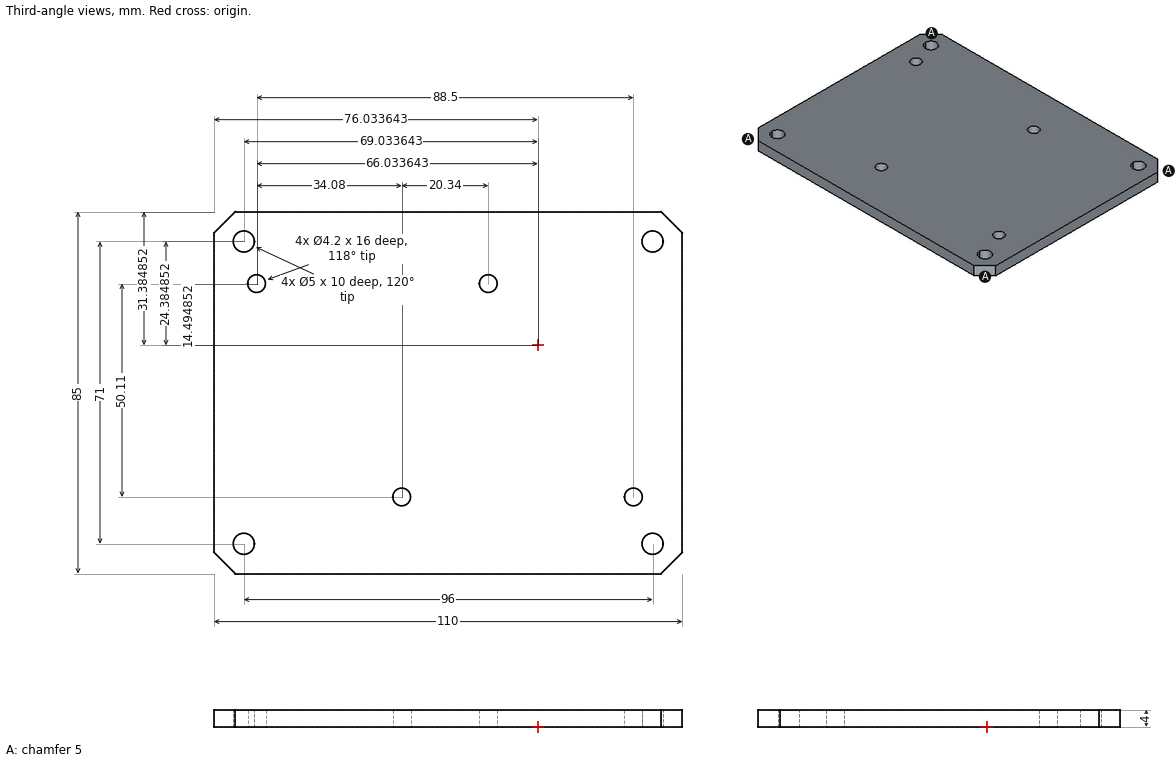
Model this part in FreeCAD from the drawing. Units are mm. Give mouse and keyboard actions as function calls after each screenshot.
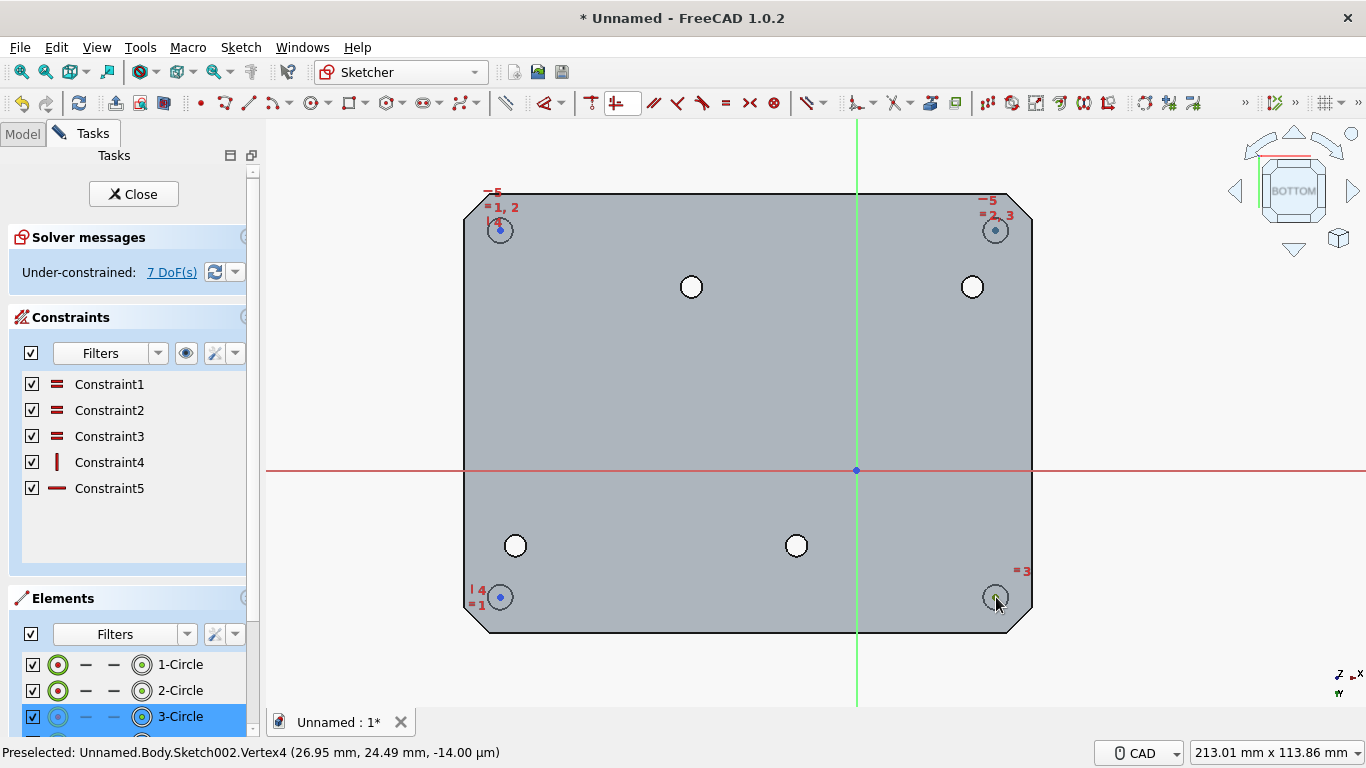
key(v)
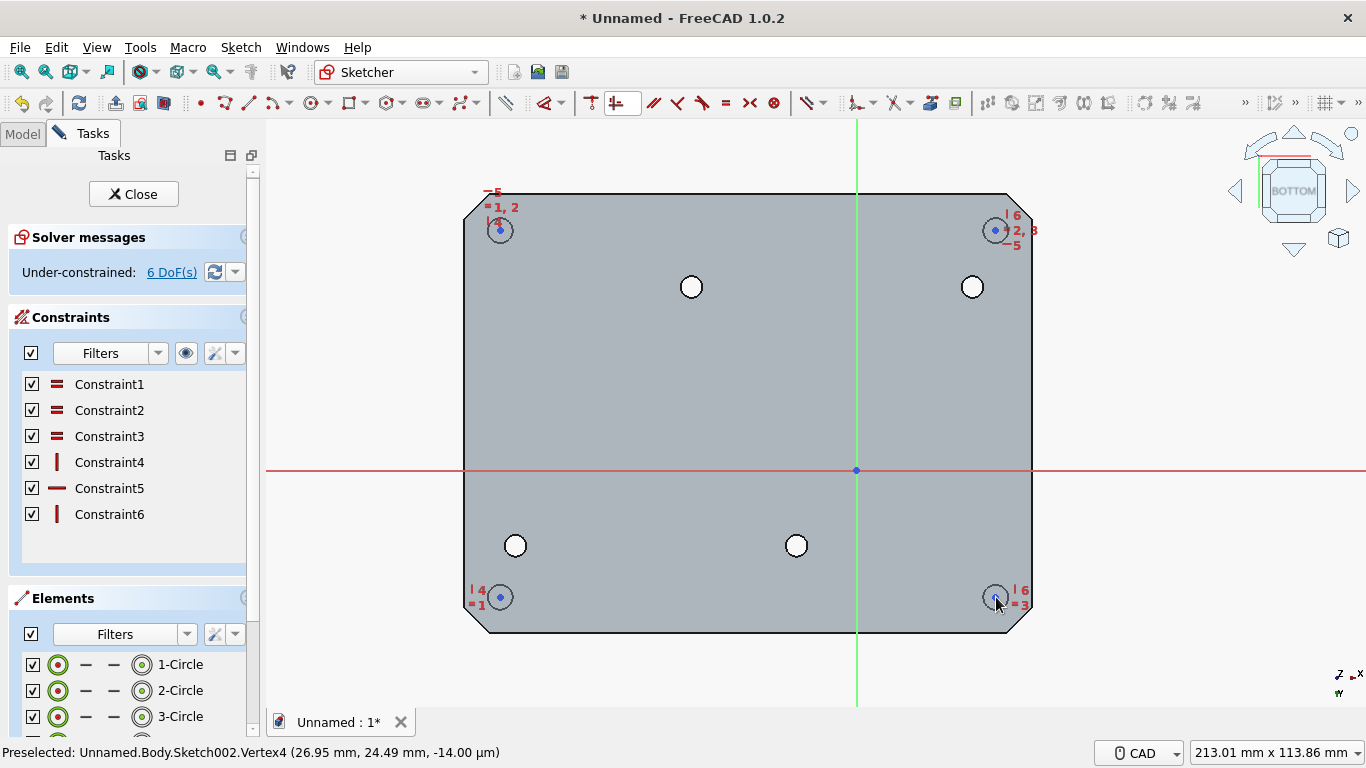
click(500, 597)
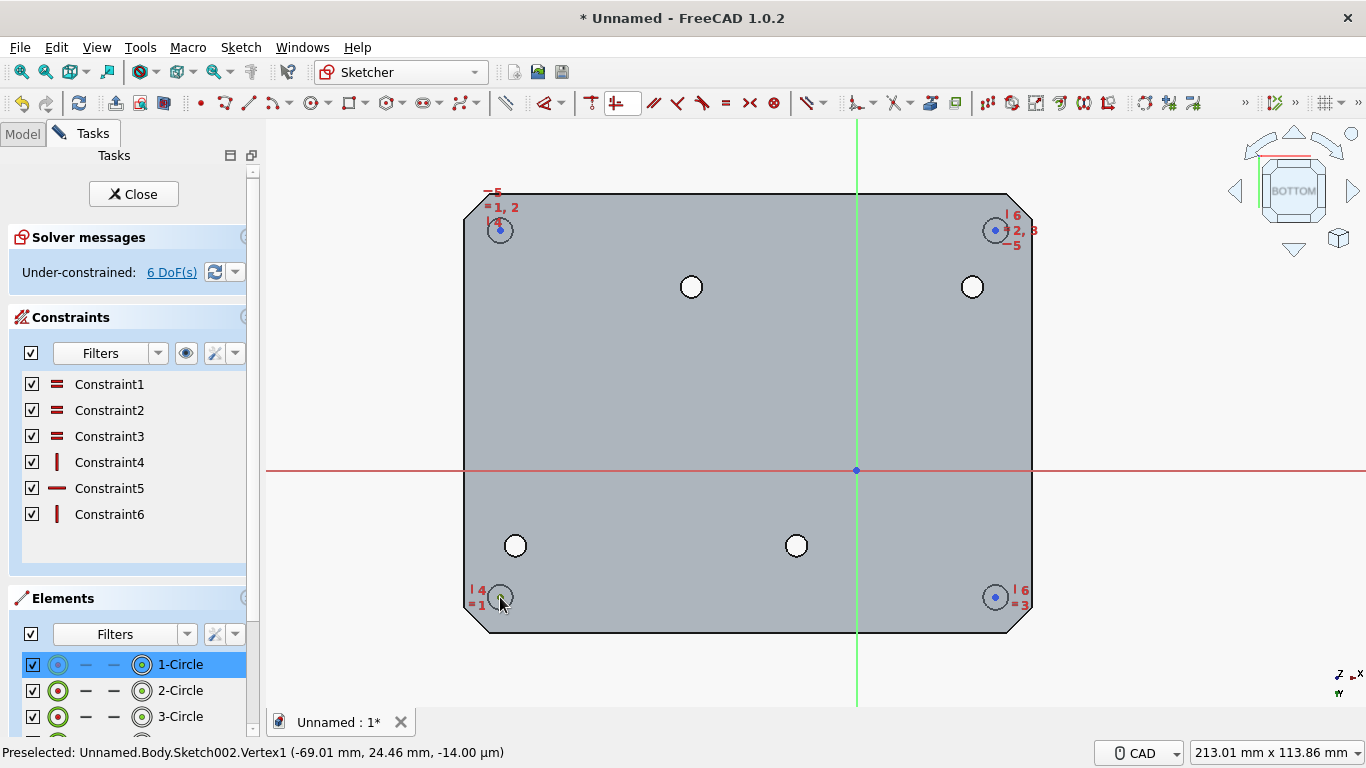
click(996, 597)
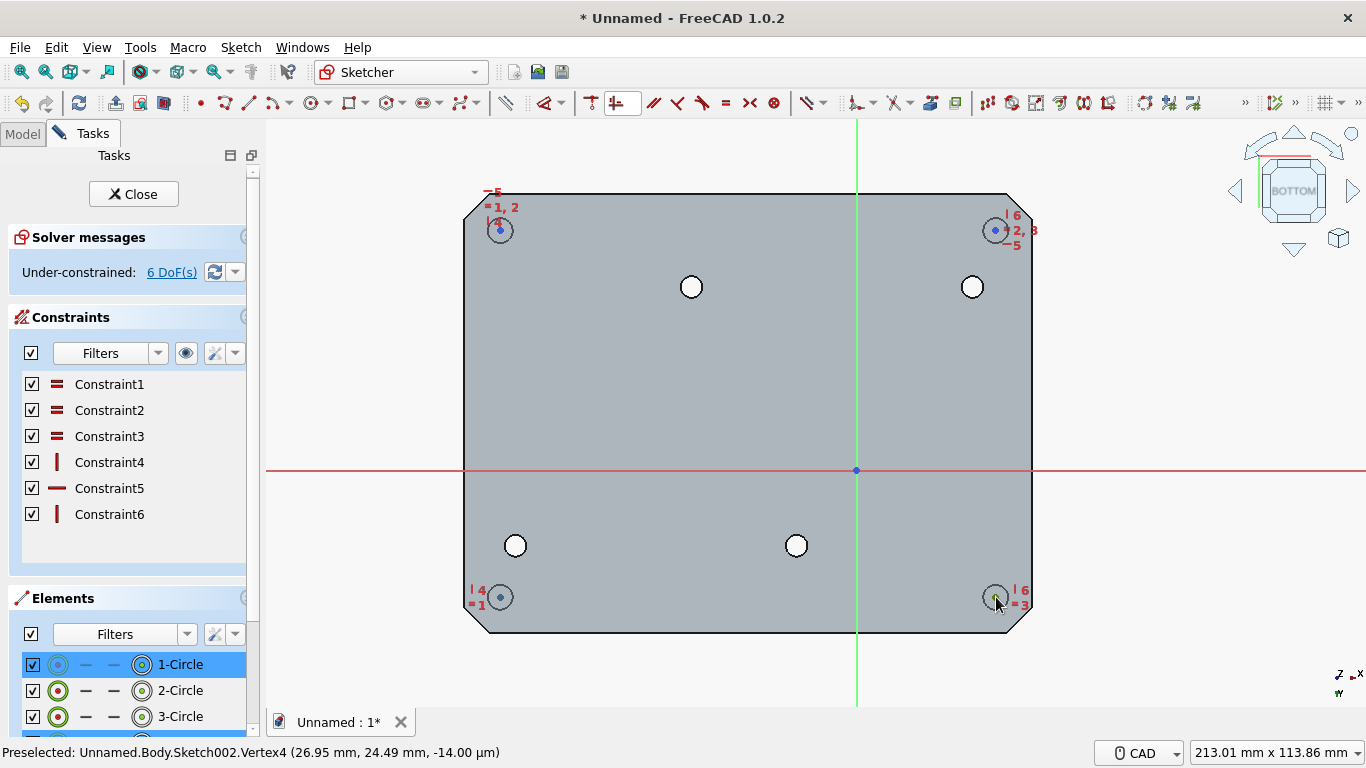
click(636, 104)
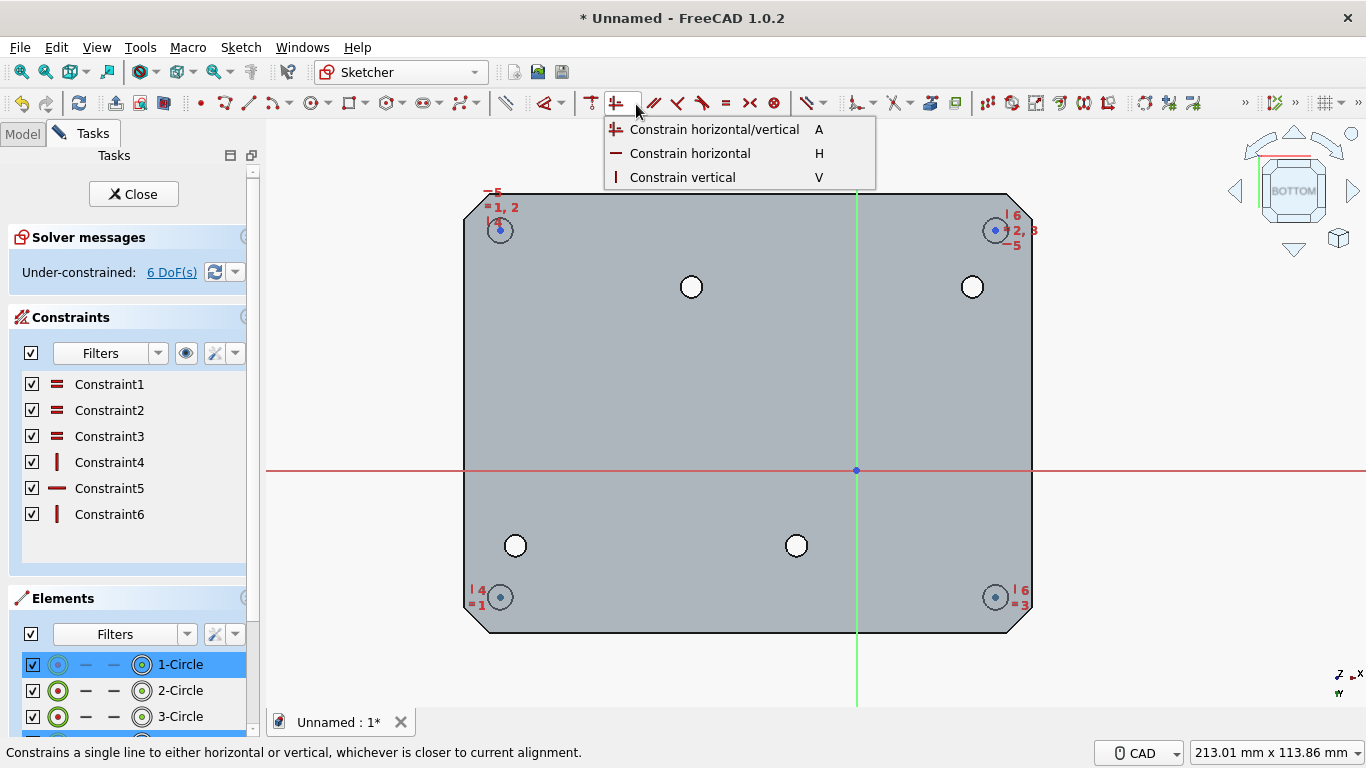
click(740, 153)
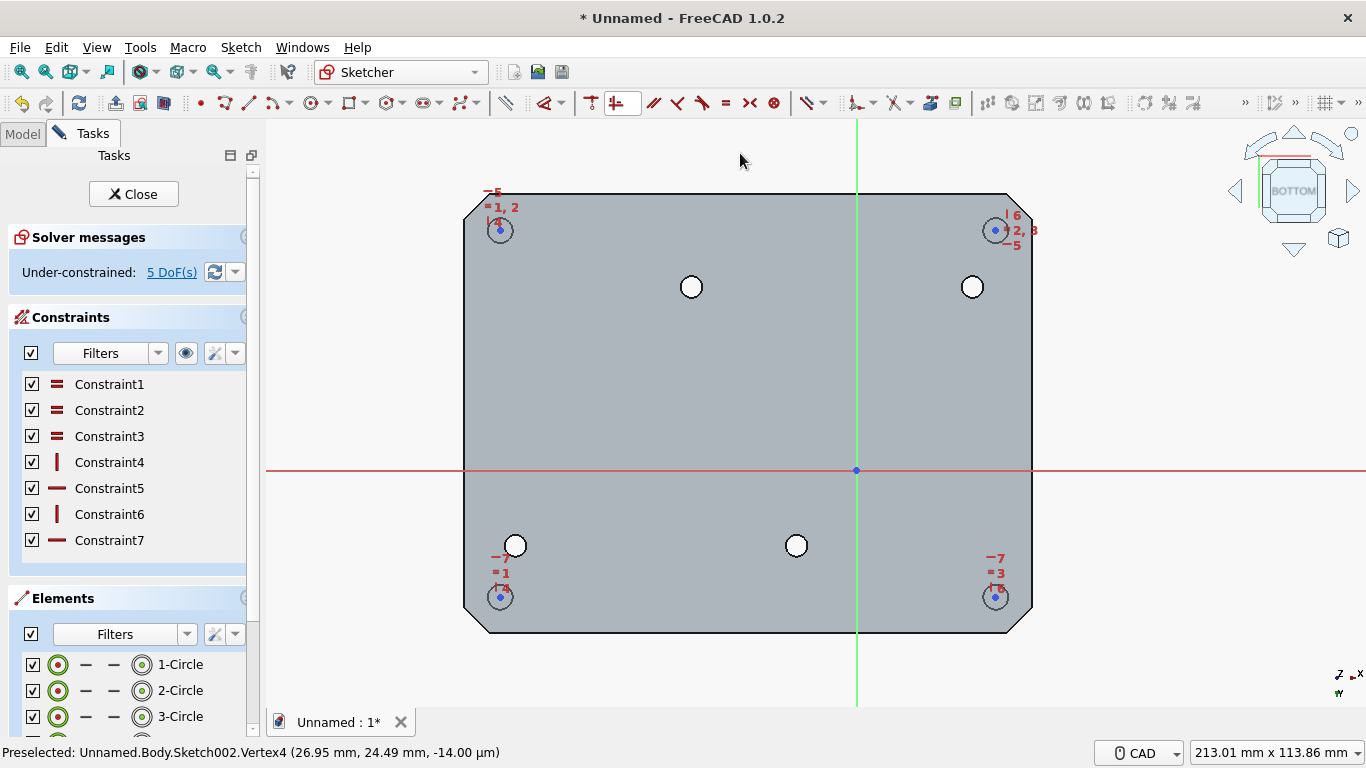
key(d)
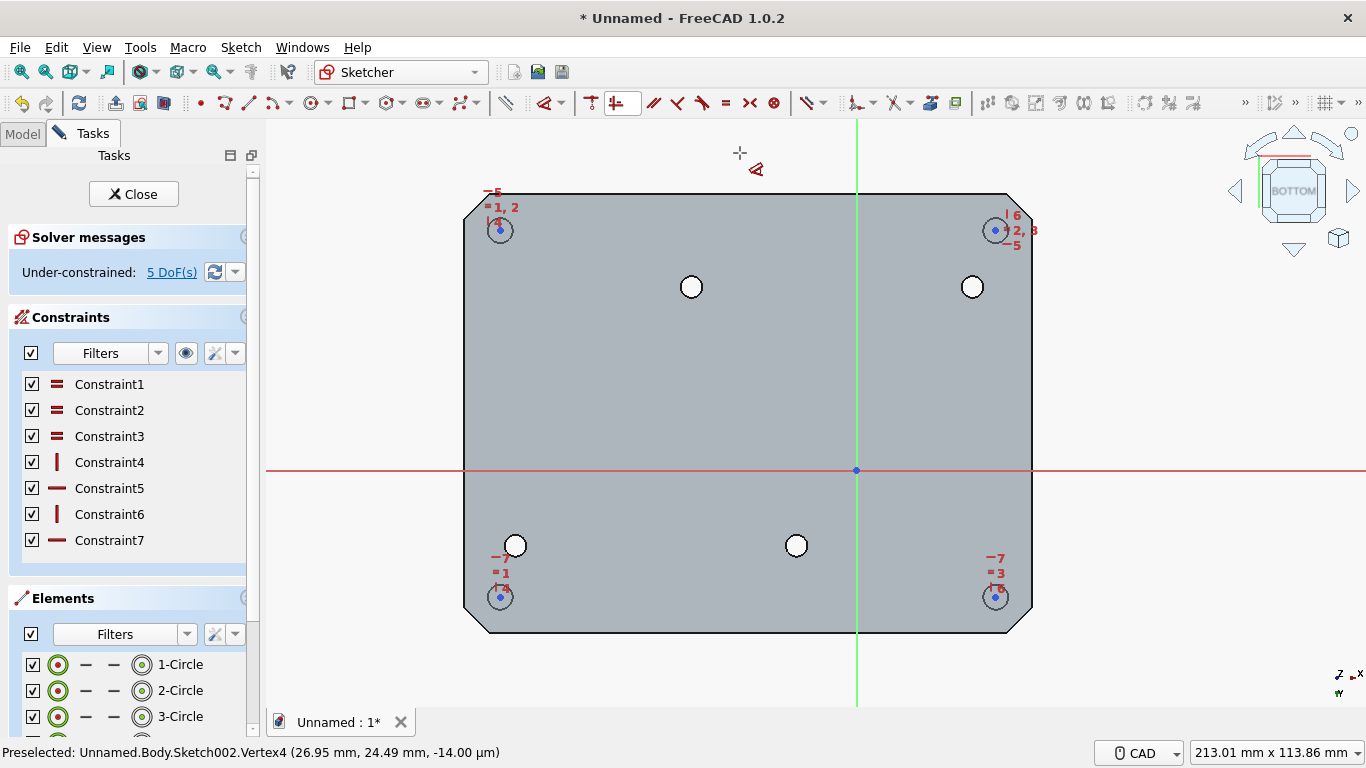
scroll(509, 588, up, 3)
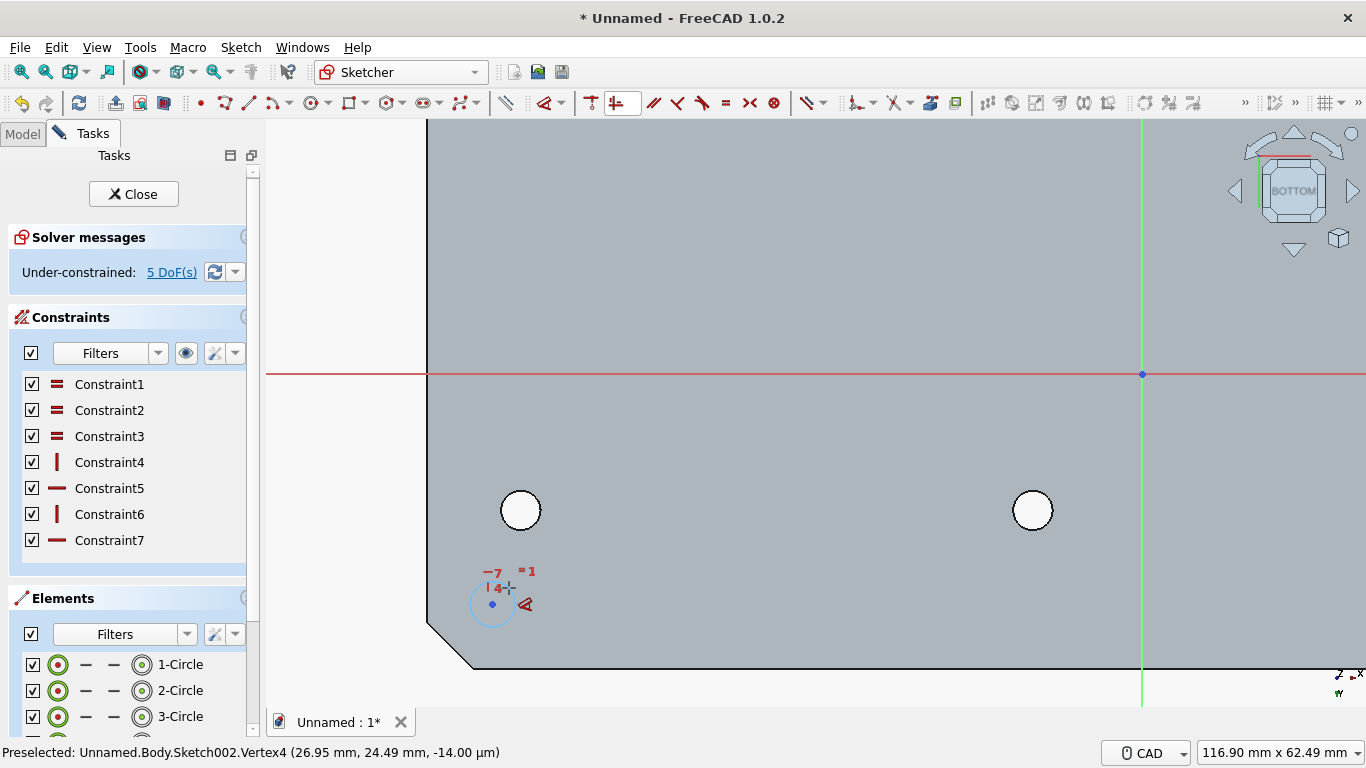
click(509, 588)
click(532, 565)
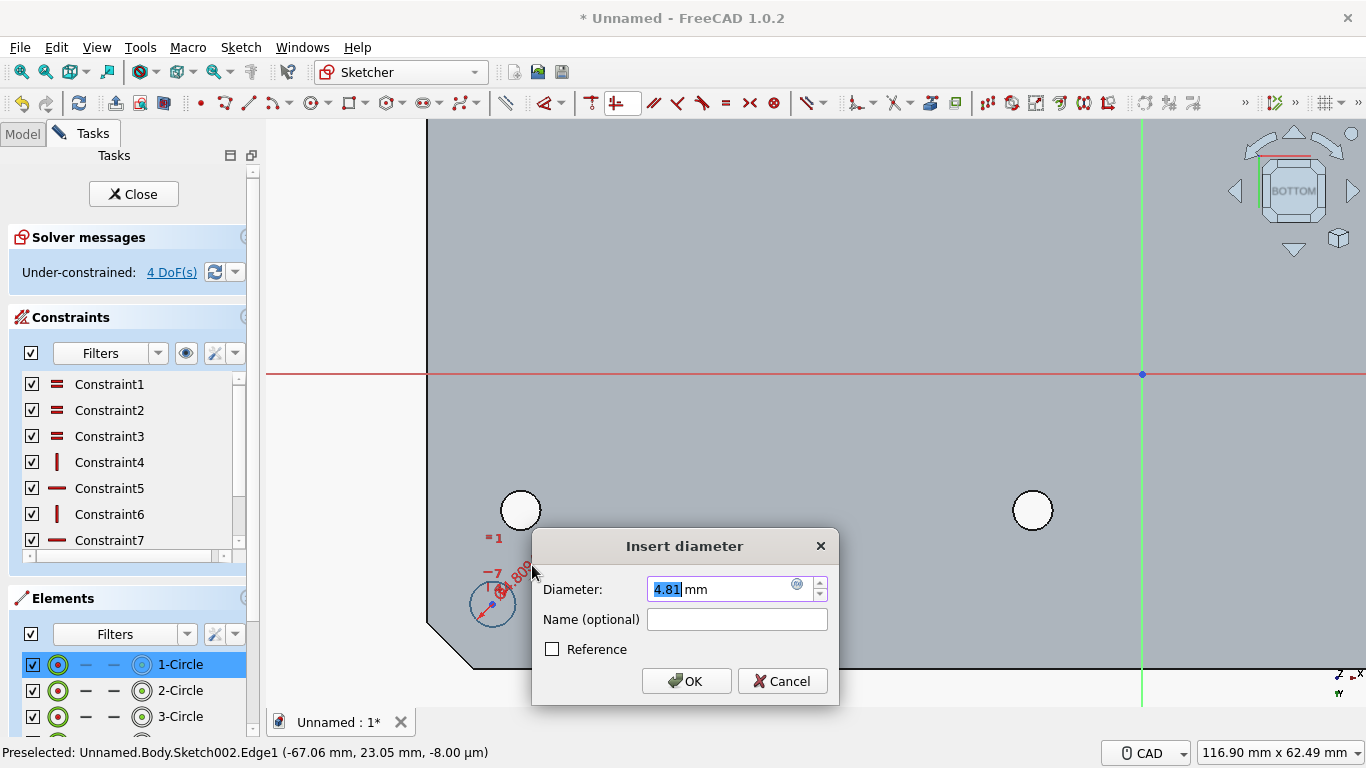
text(5)
key(Return)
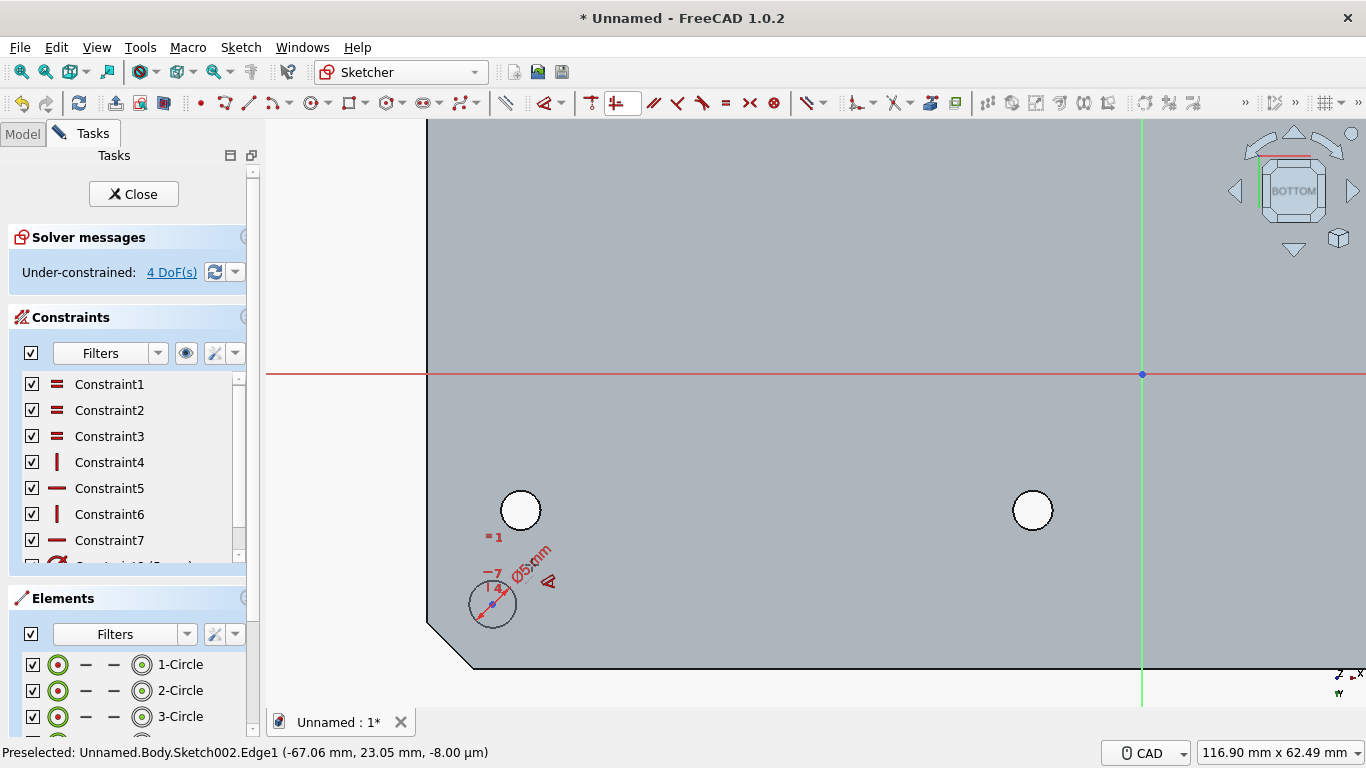
click(493, 604)